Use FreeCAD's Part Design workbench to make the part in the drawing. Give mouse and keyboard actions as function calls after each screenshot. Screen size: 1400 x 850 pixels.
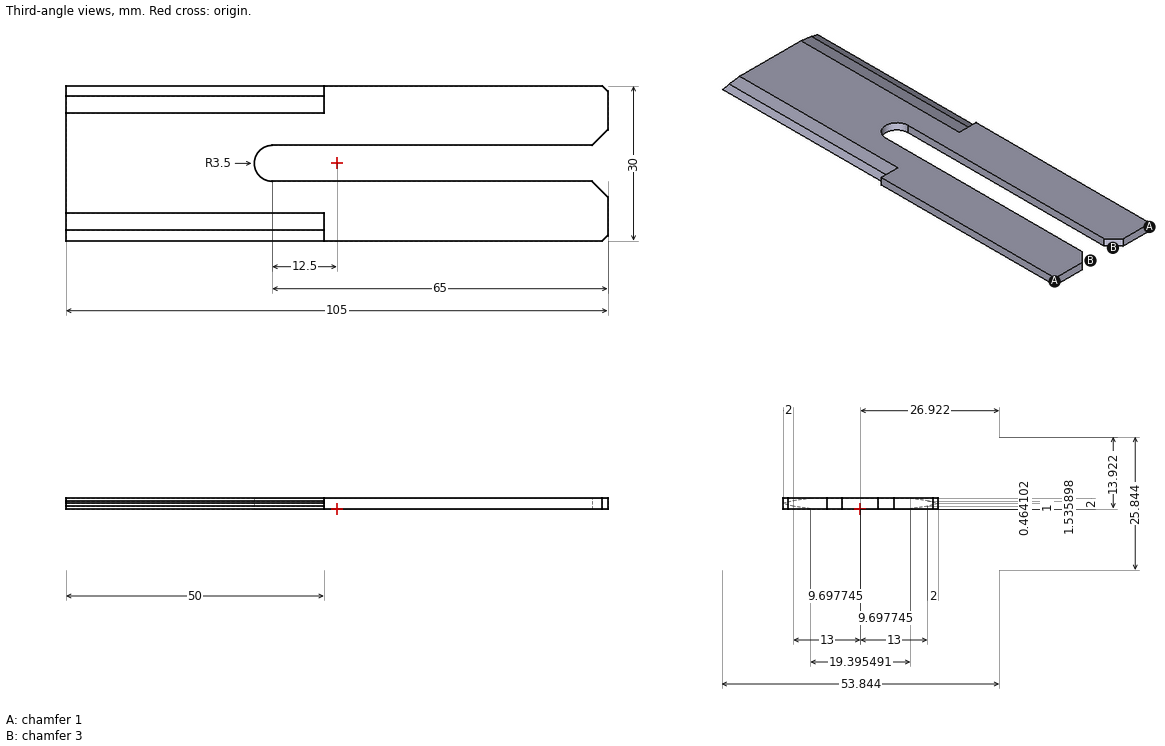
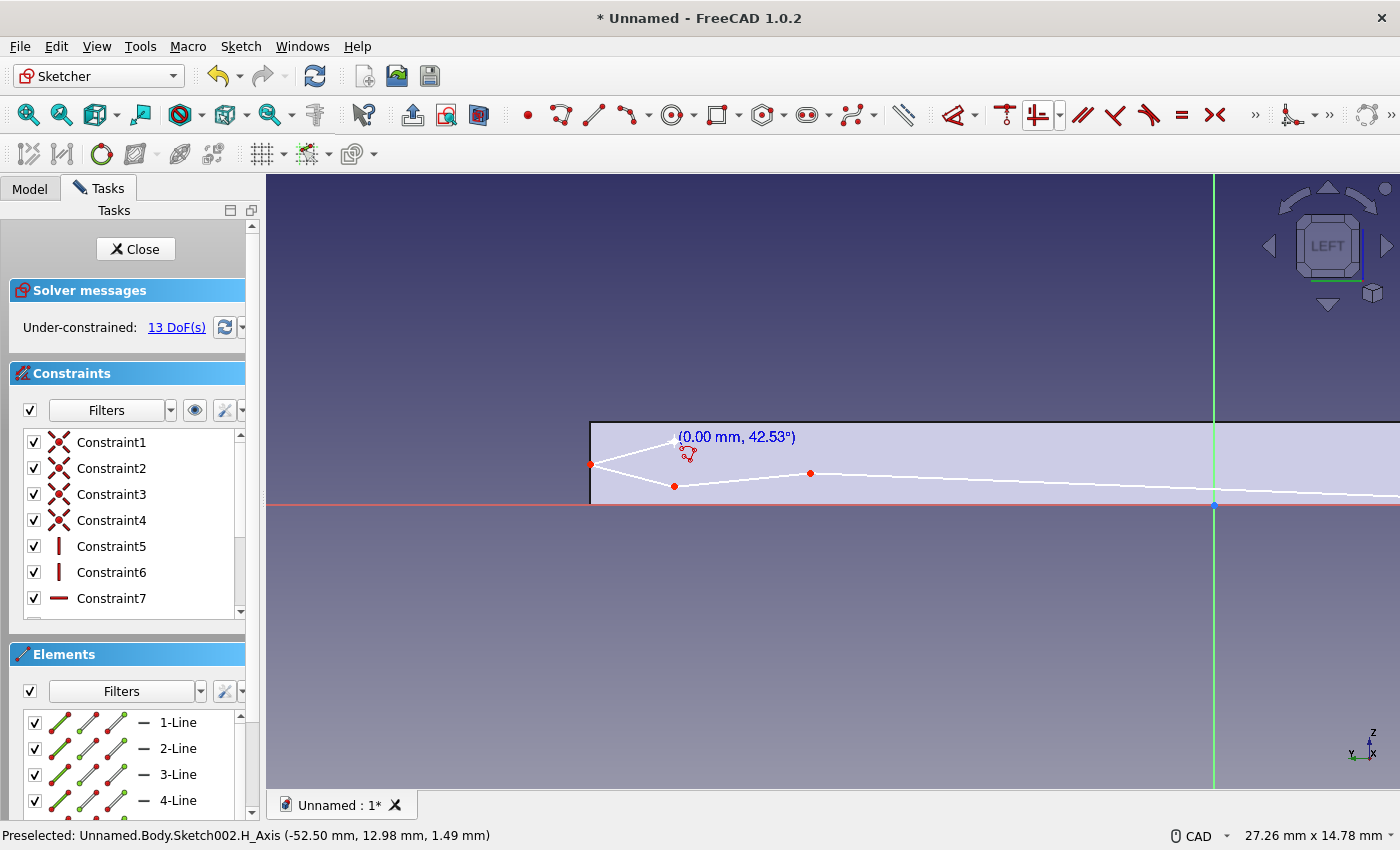
scroll(571, 489, down, 6)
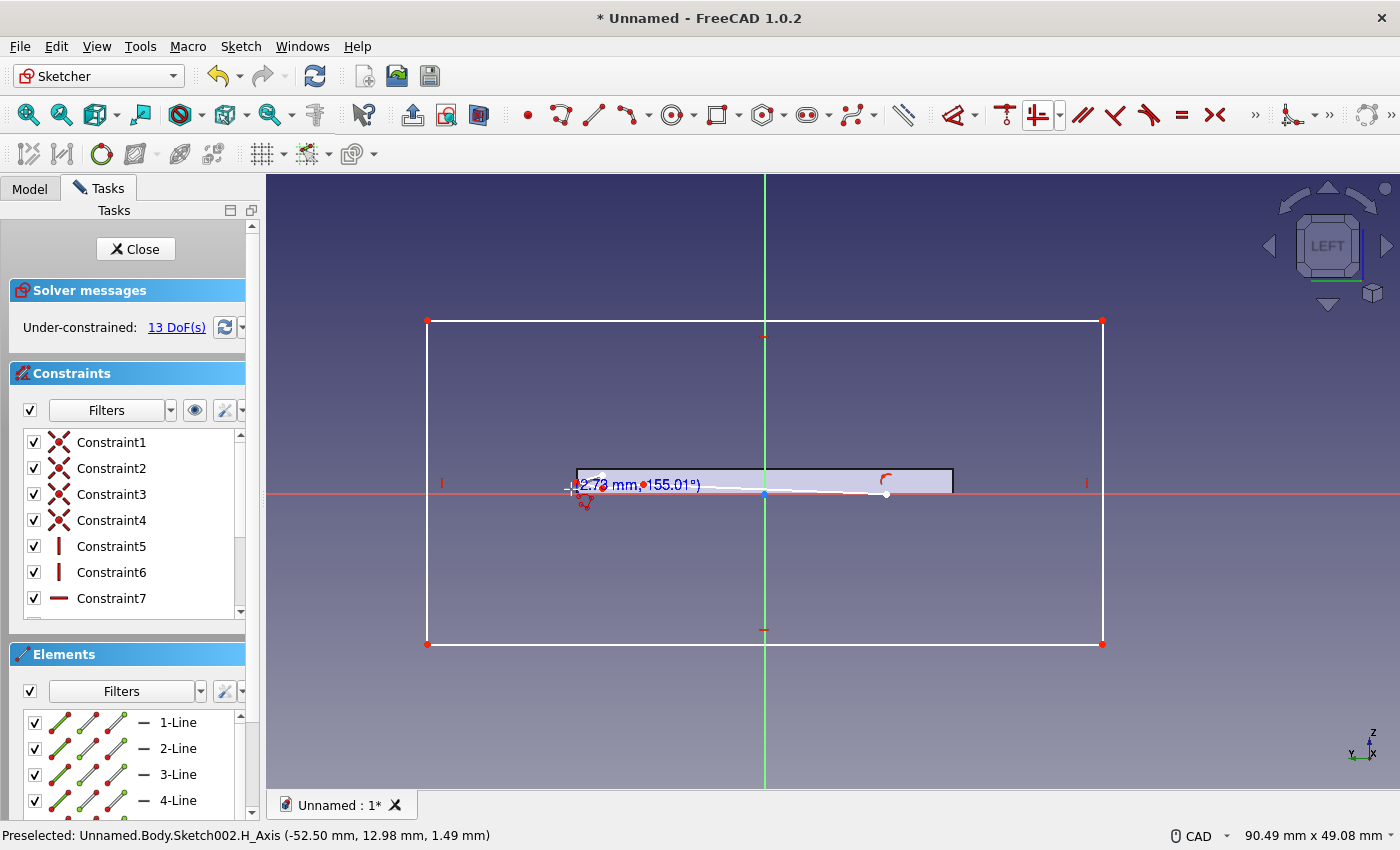
click(643, 469)
click(887, 469)
click(928, 475)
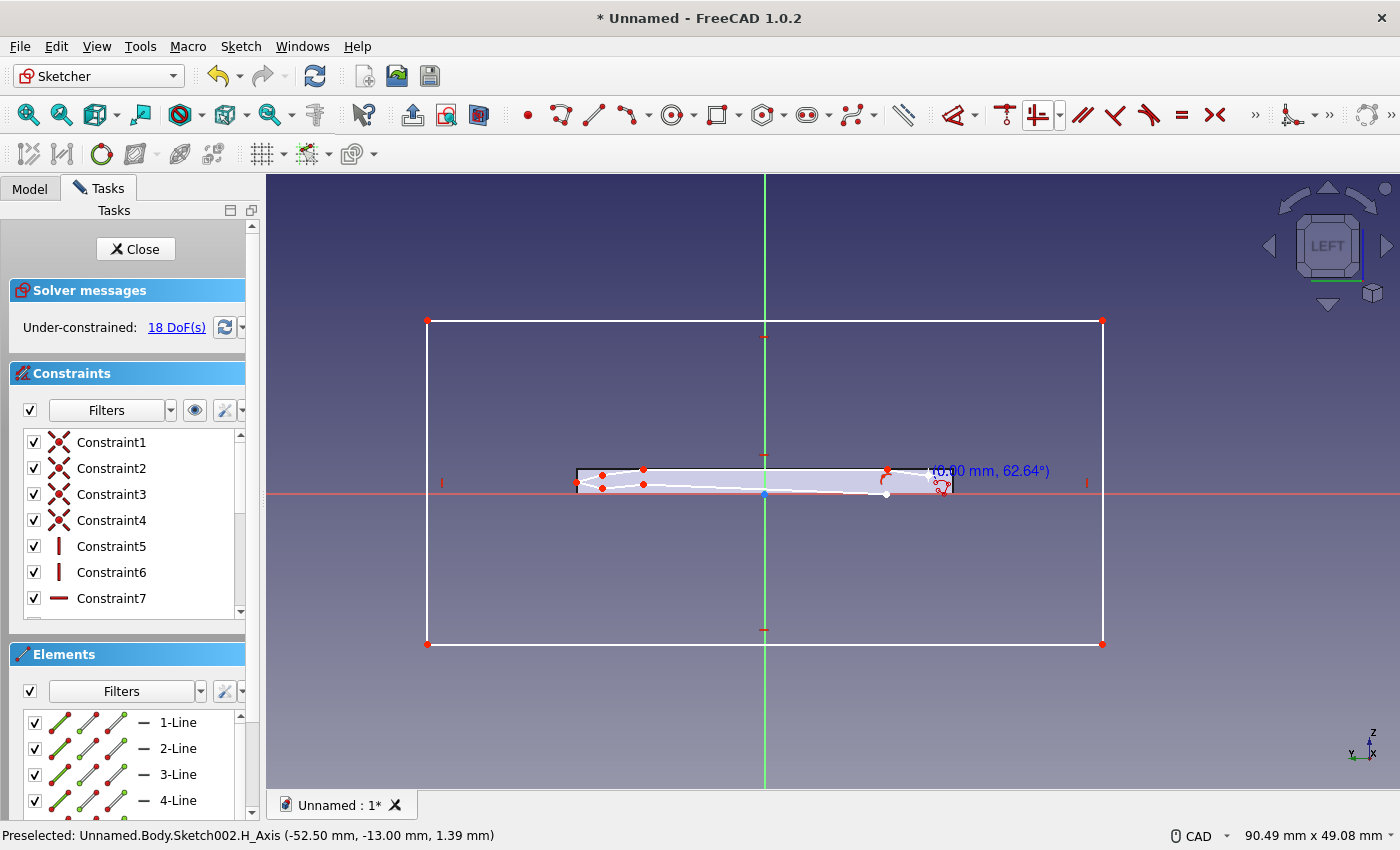
scroll(953, 482, up, 2)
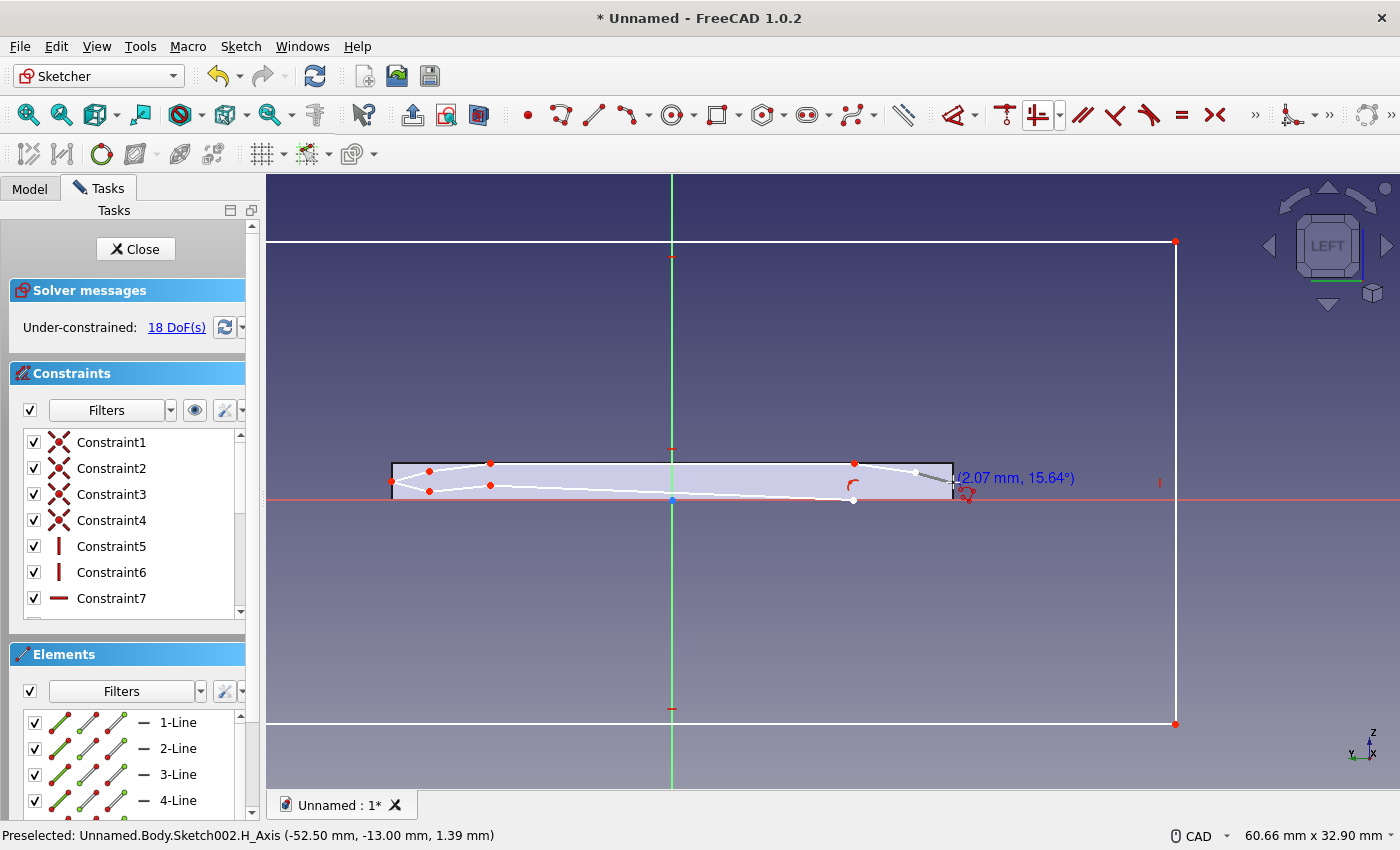
click(953, 481)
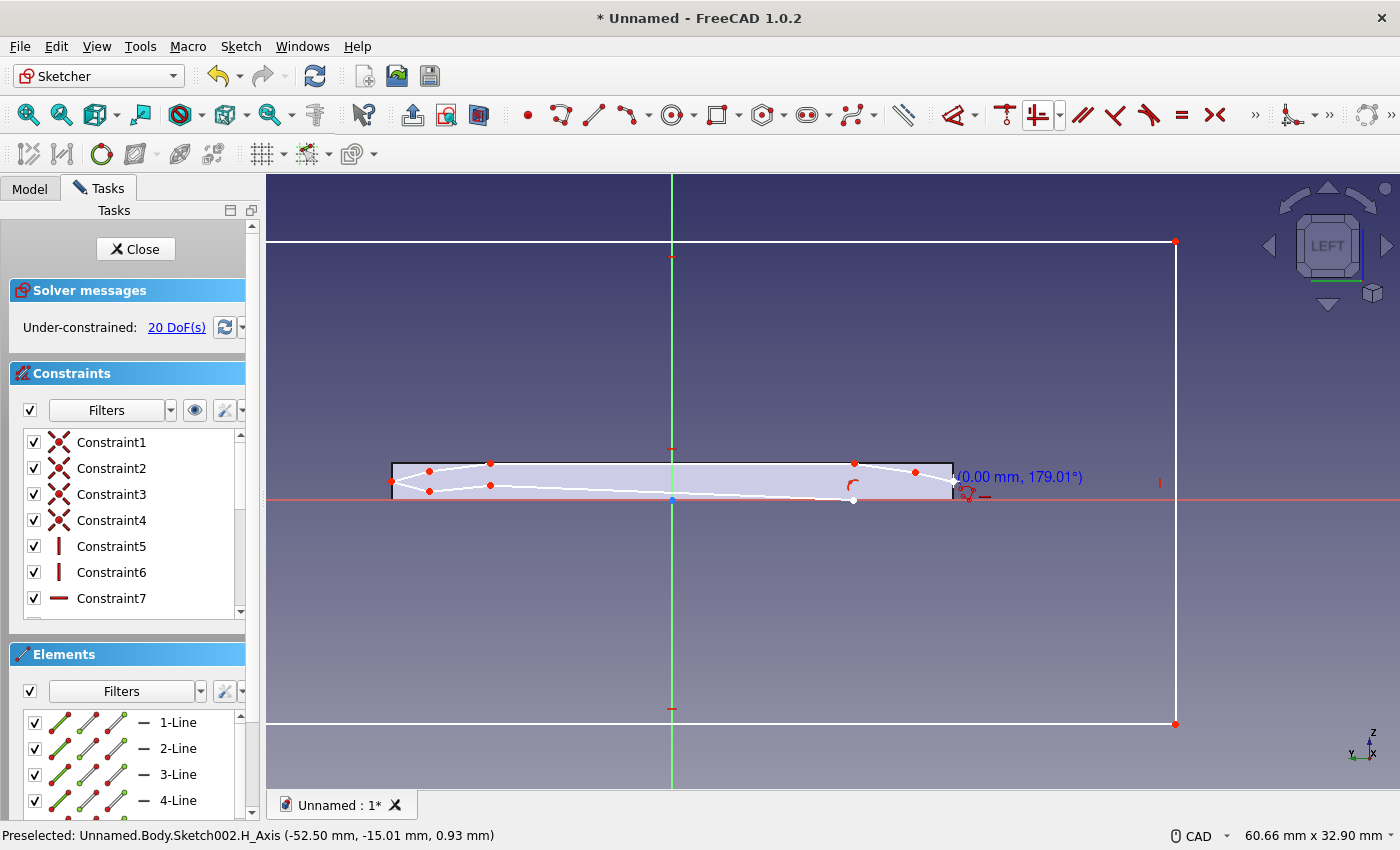
scroll(915, 491, up, 4)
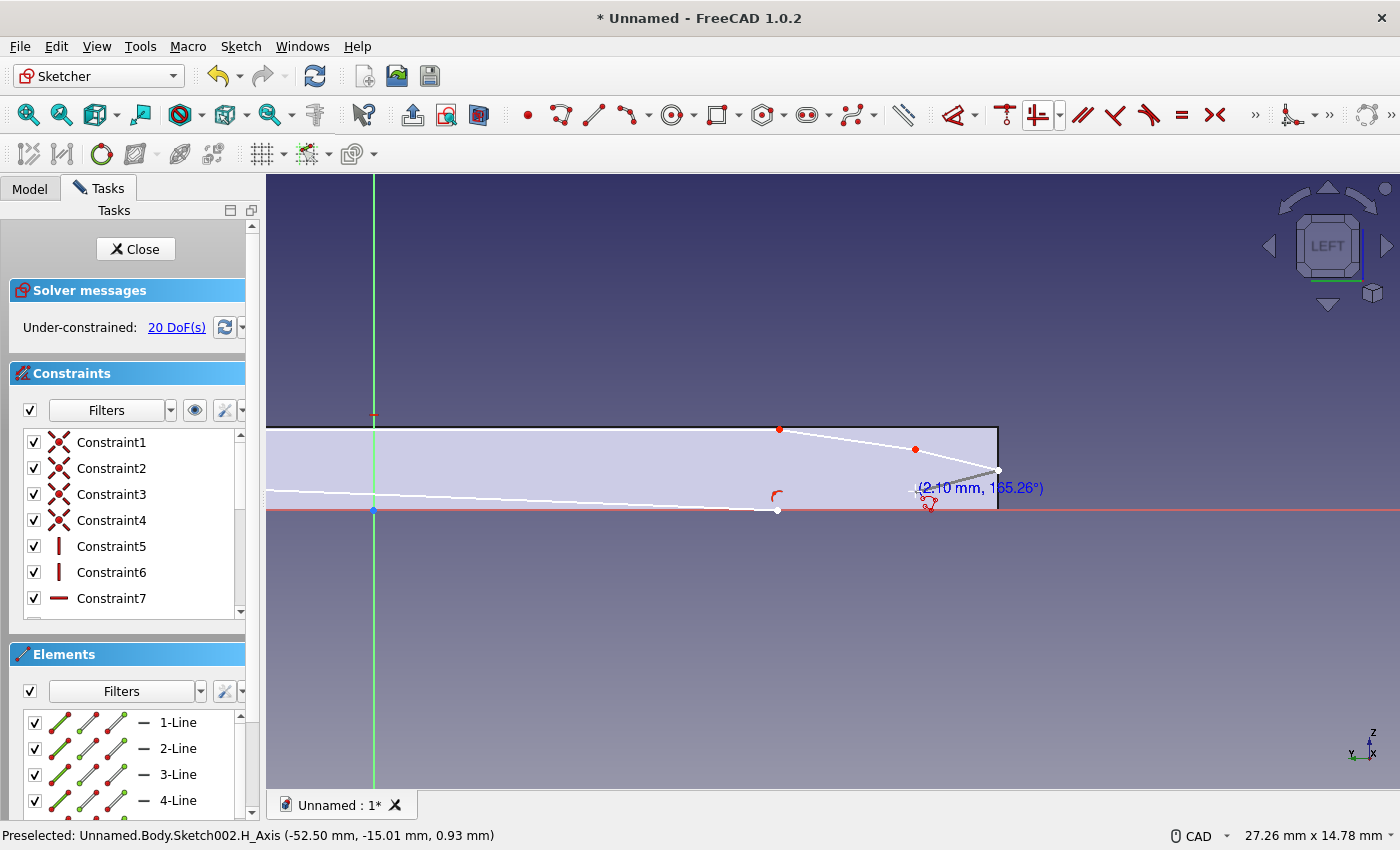
click(915, 491)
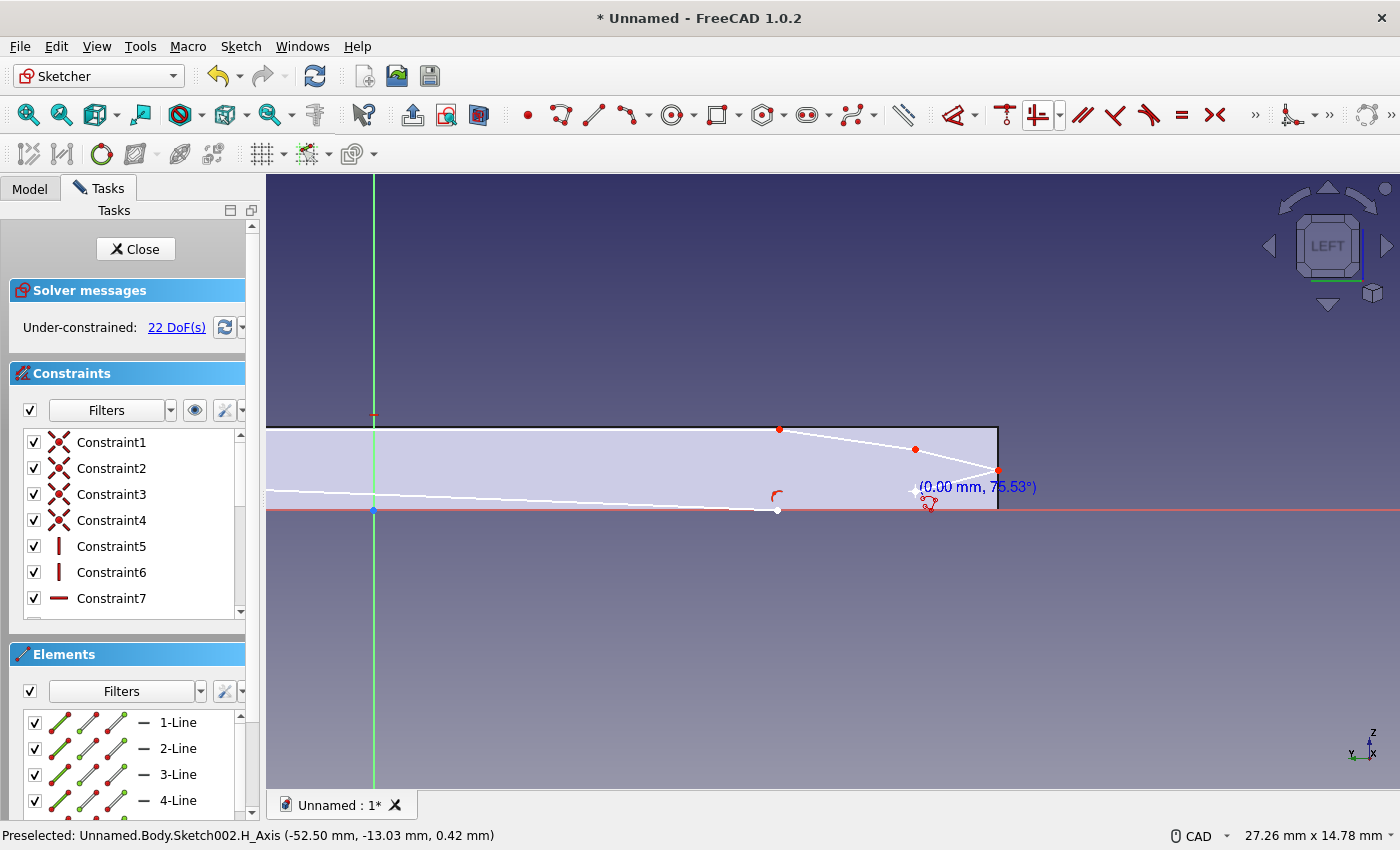
scroll(933, 487, down, 6)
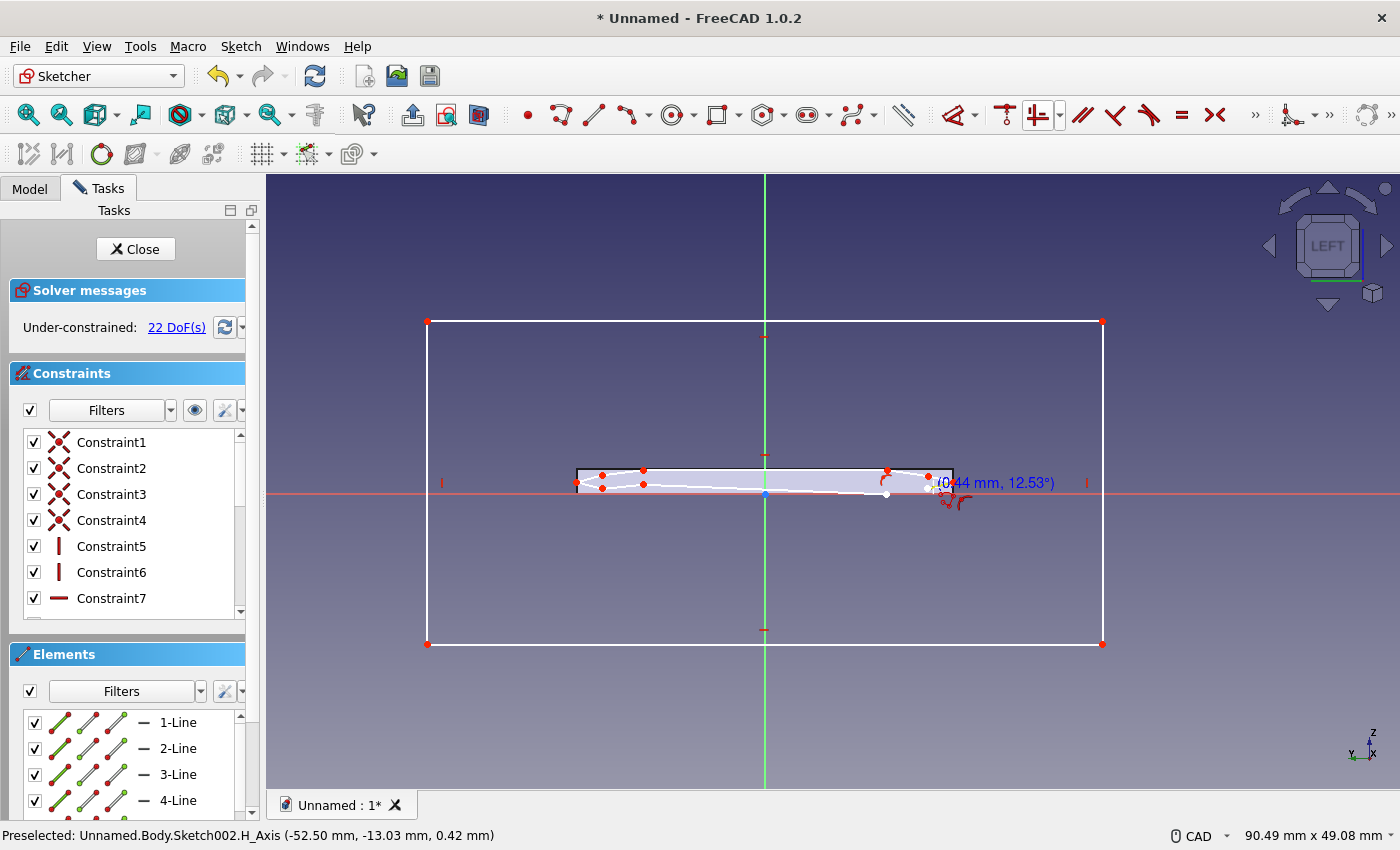
click(887, 494)
key(Escape)
key(Escape)